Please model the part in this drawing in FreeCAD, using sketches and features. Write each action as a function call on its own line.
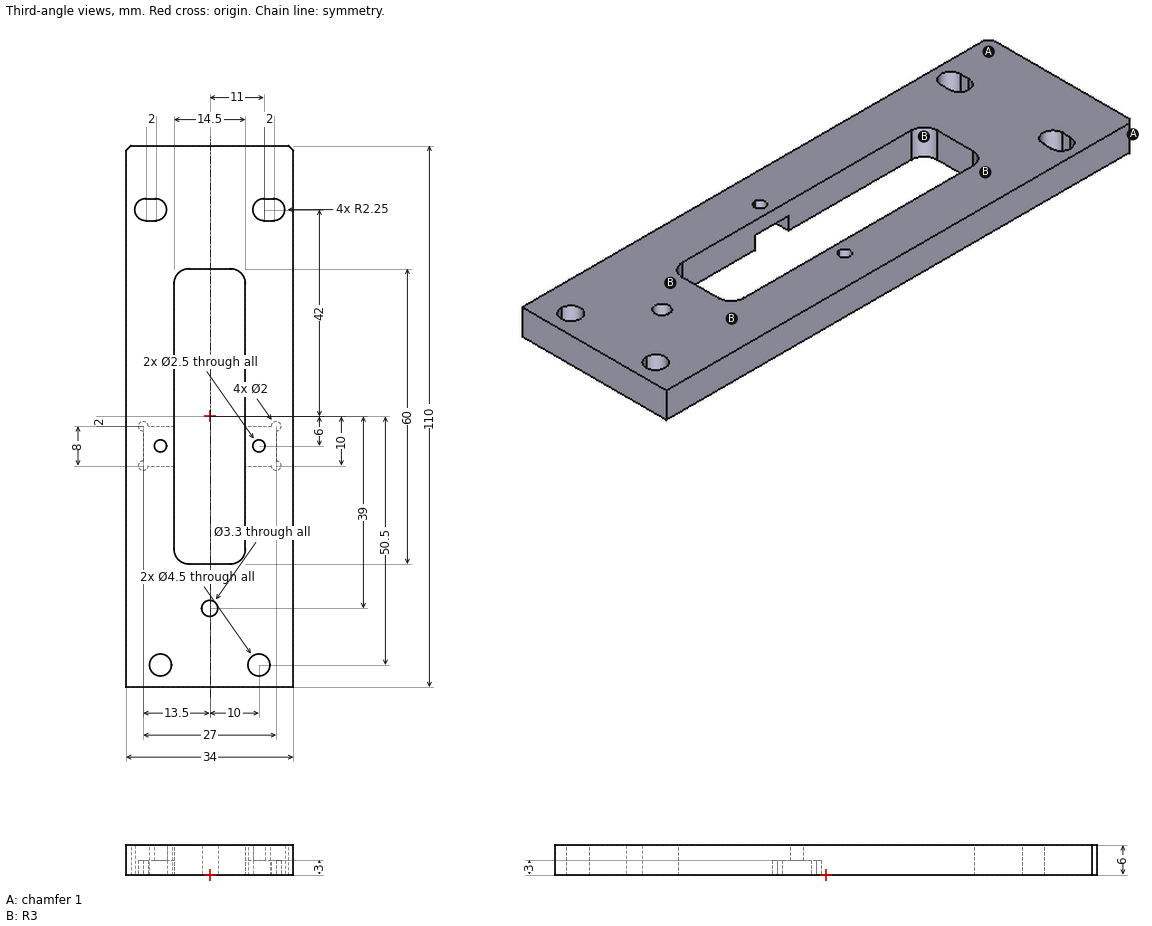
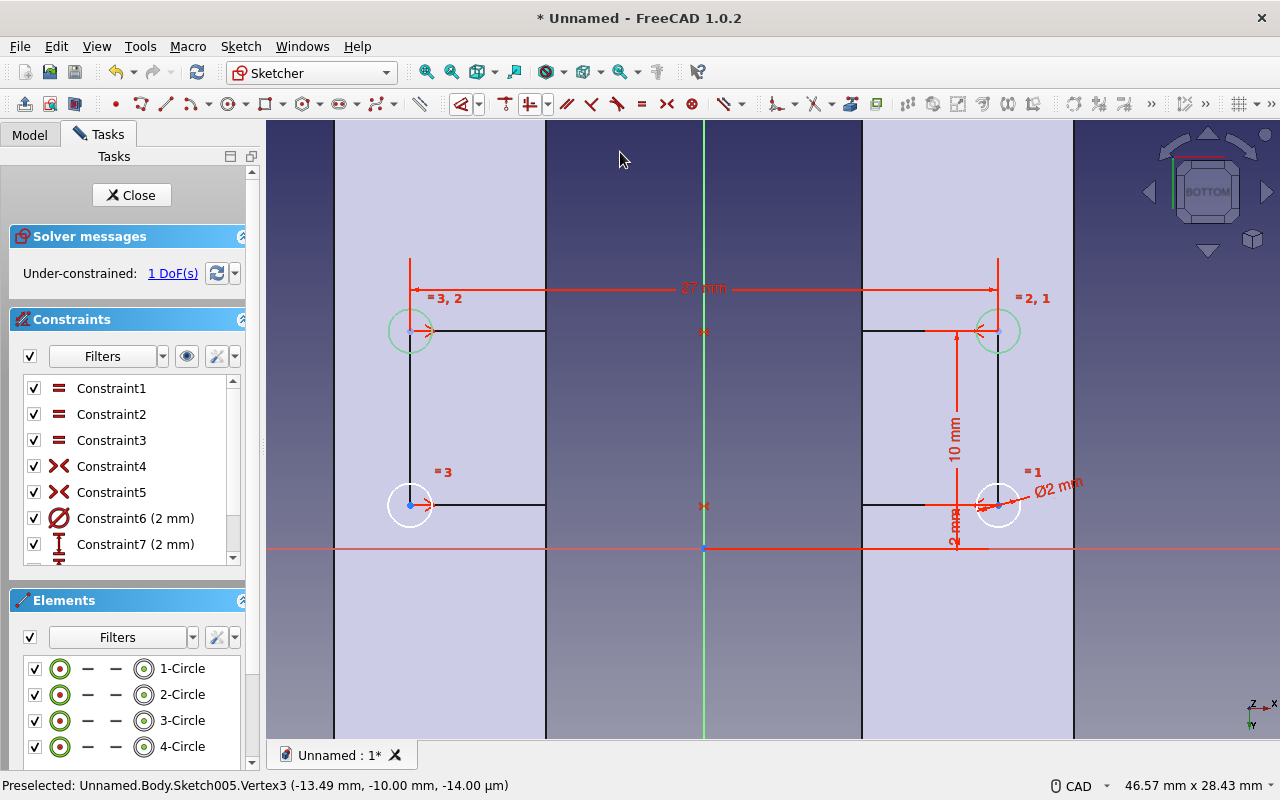
click(998, 505)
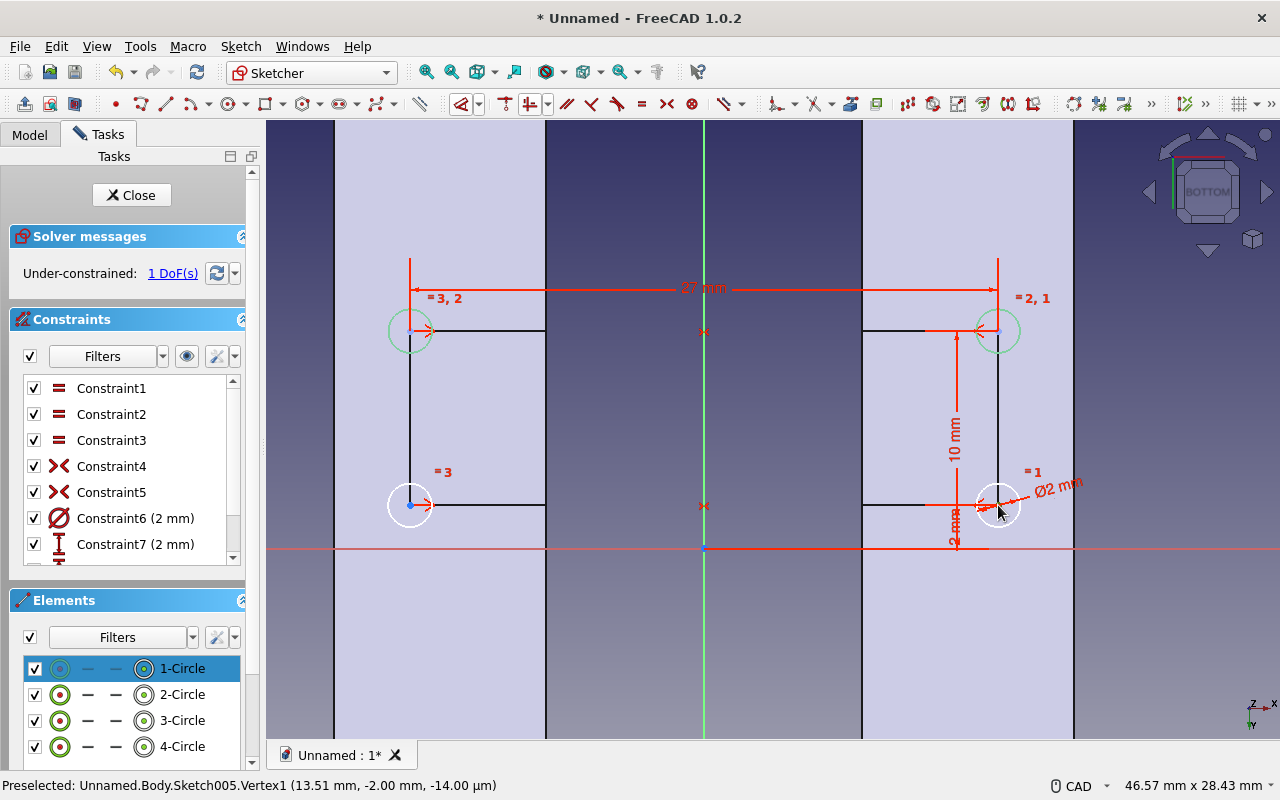
click(410, 331)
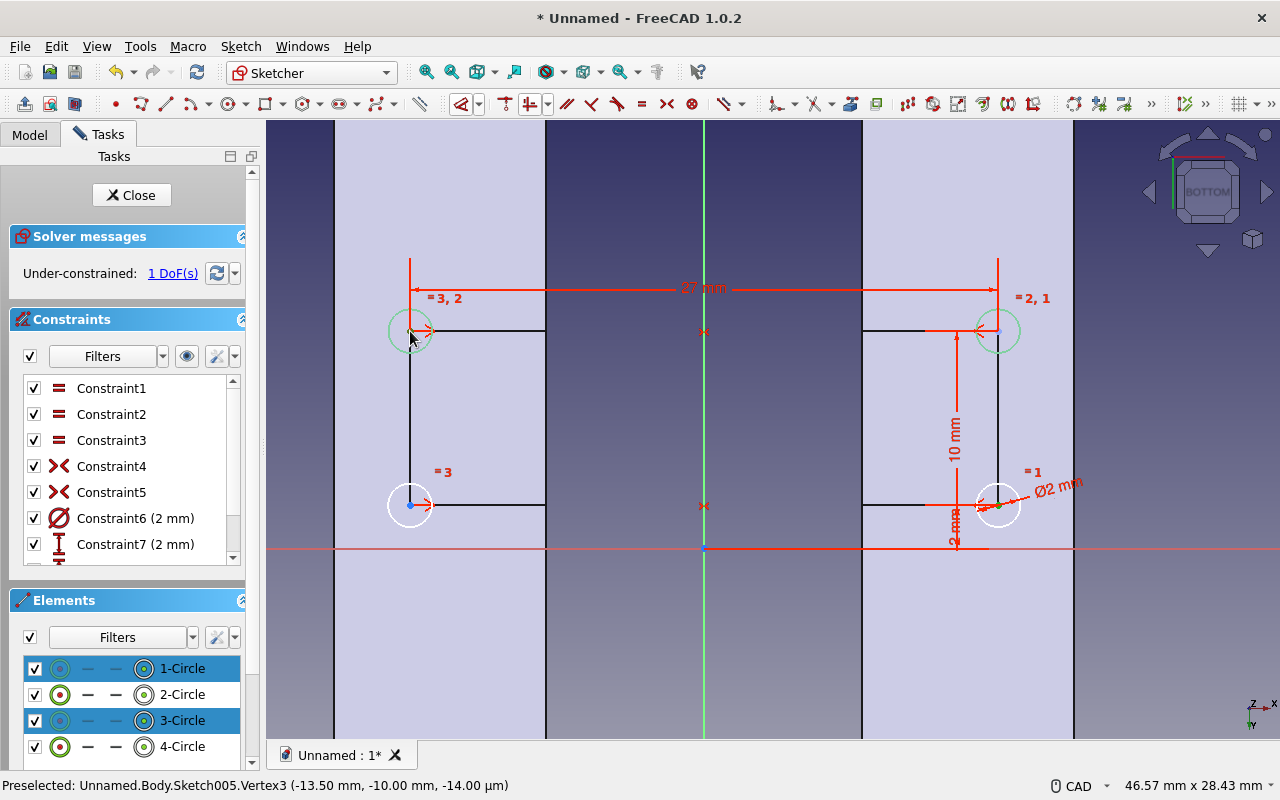
click(478, 104)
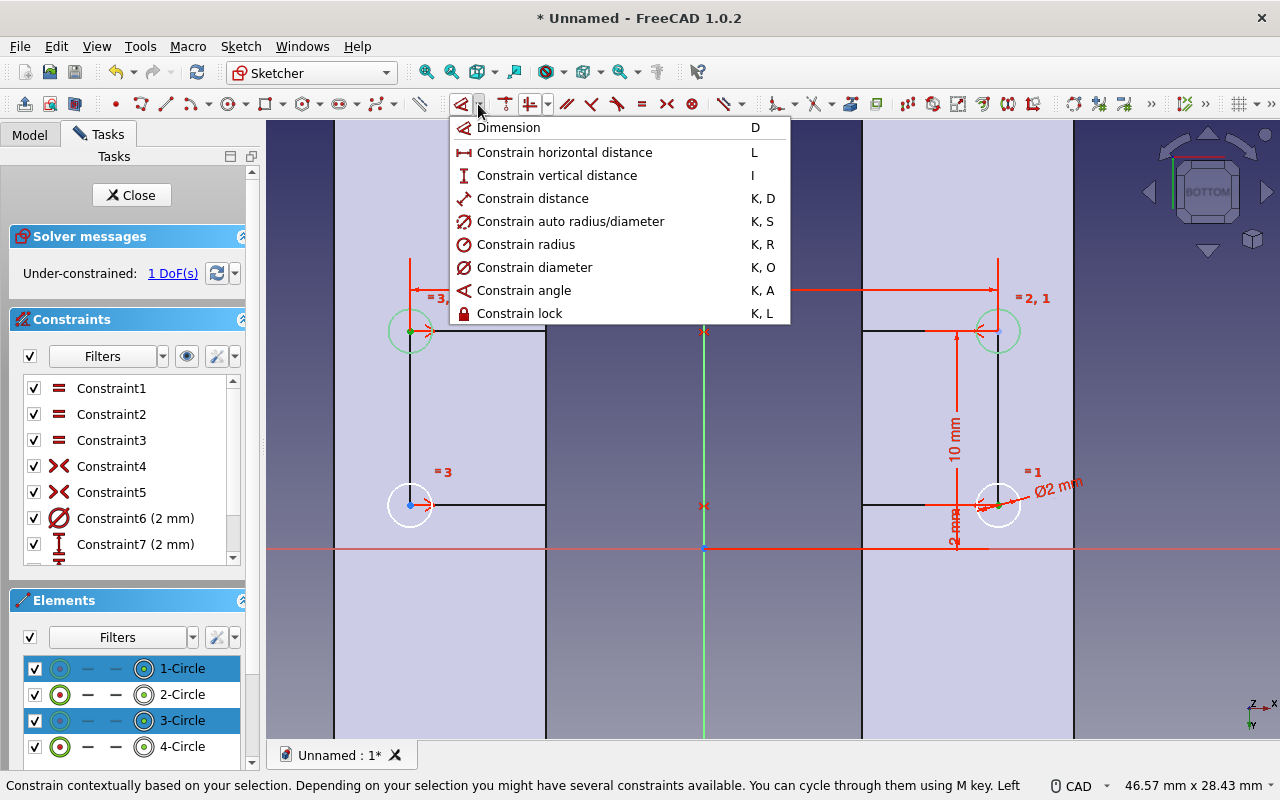
click(620, 152)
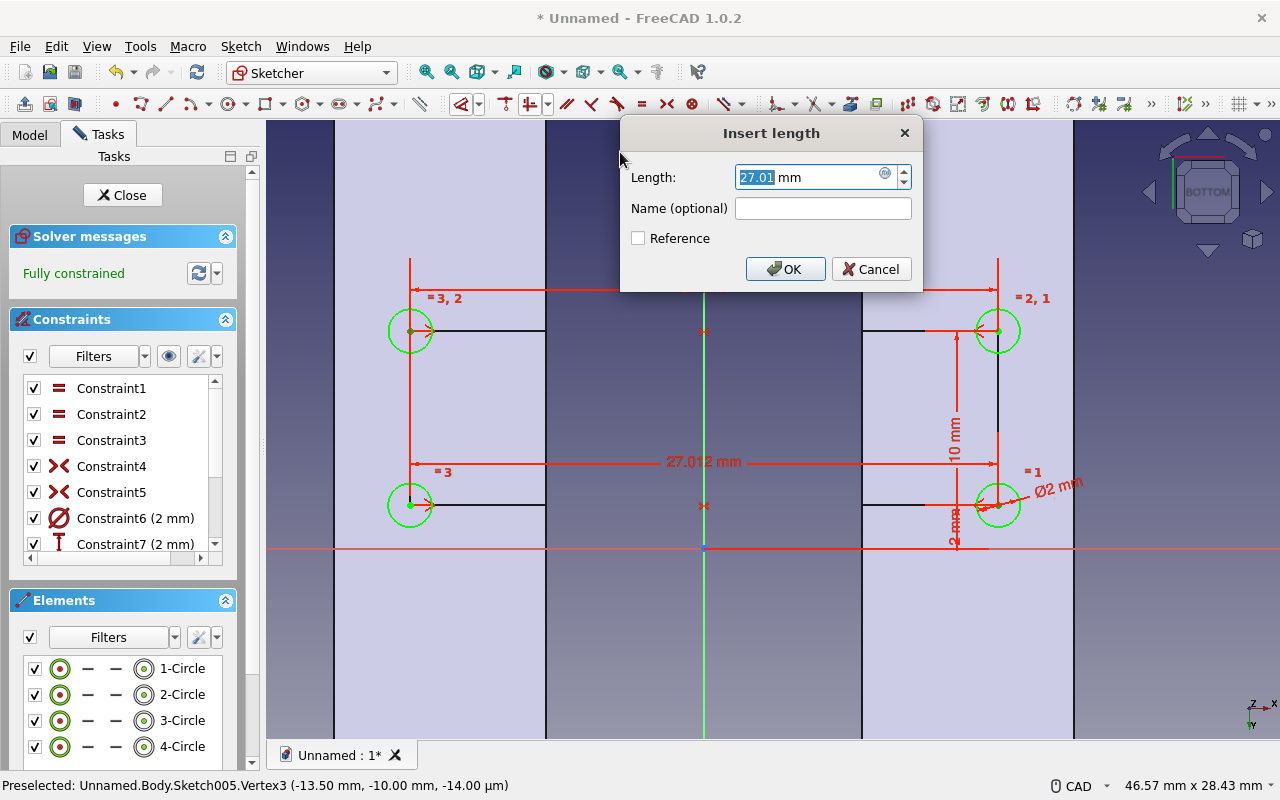
text(27)
key(Return)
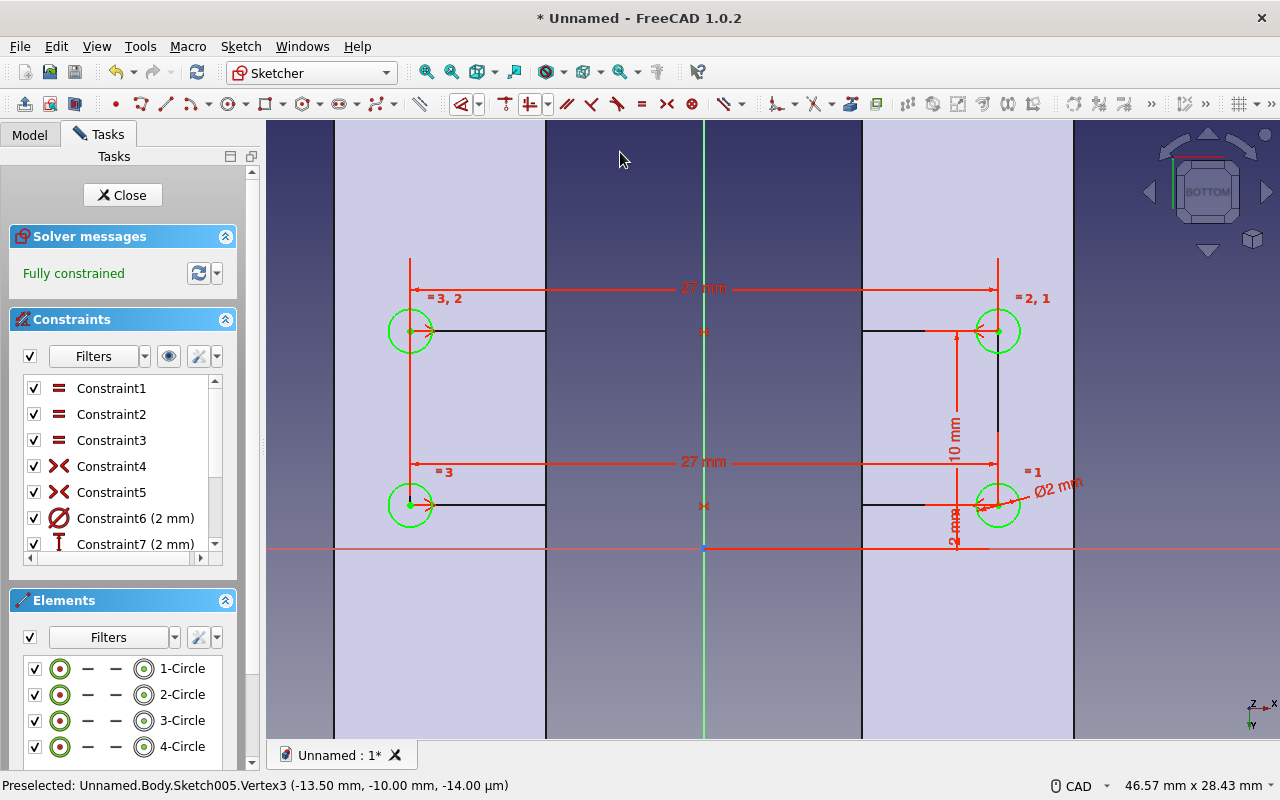
click(123, 195)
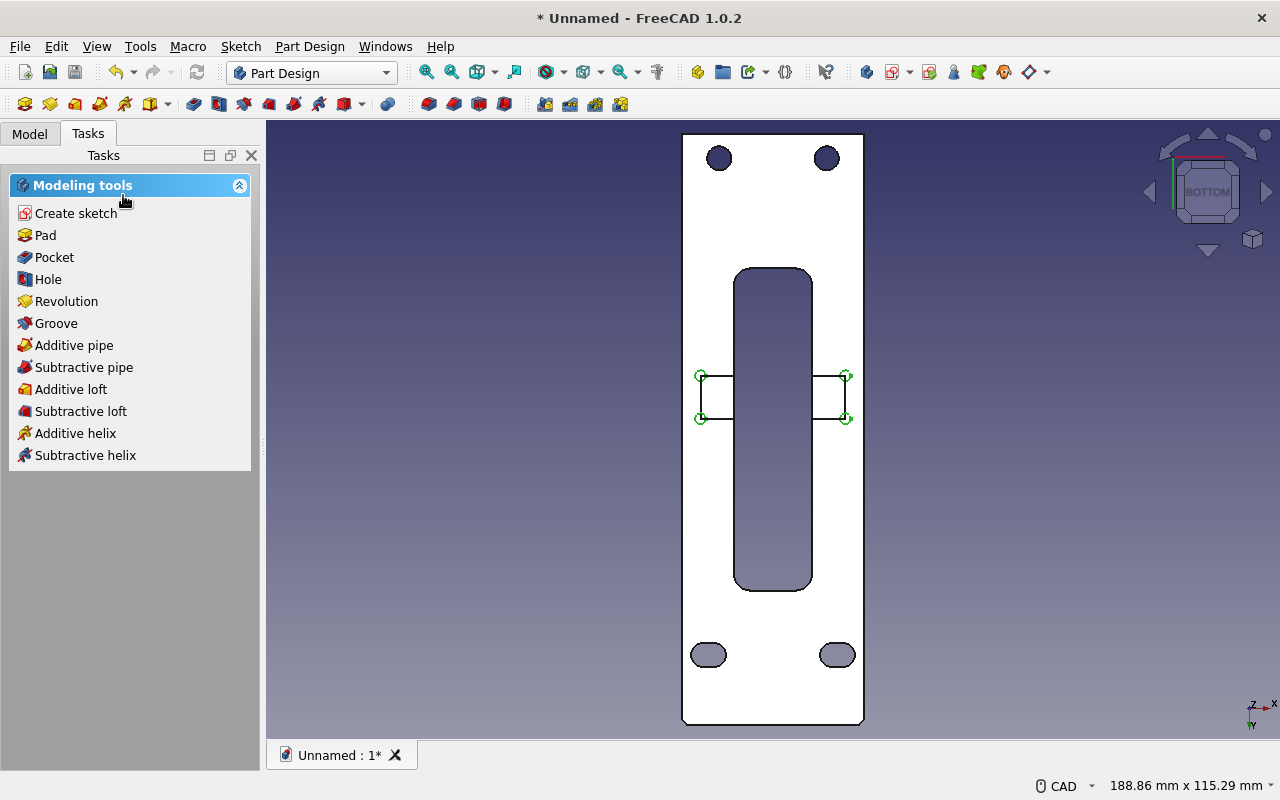
click(194, 104)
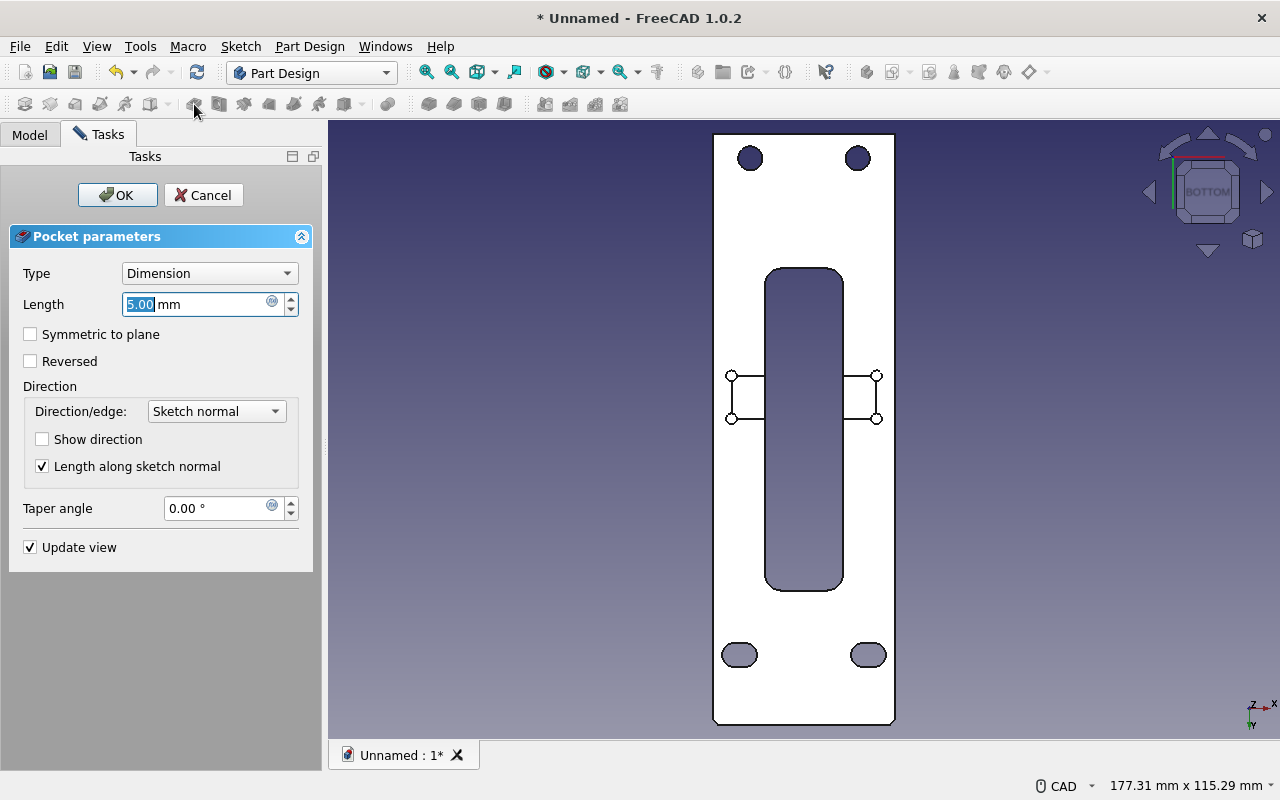
text(3)
key(Tab)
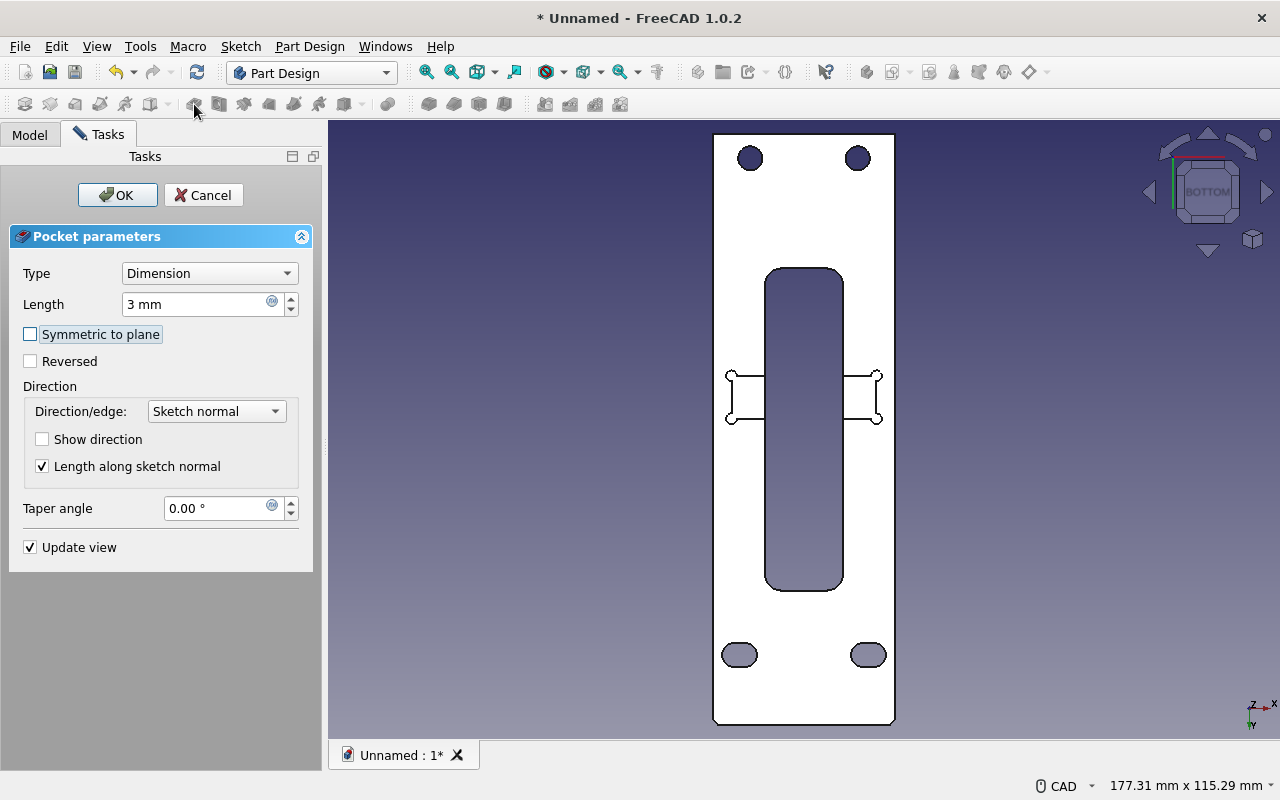
click(118, 195)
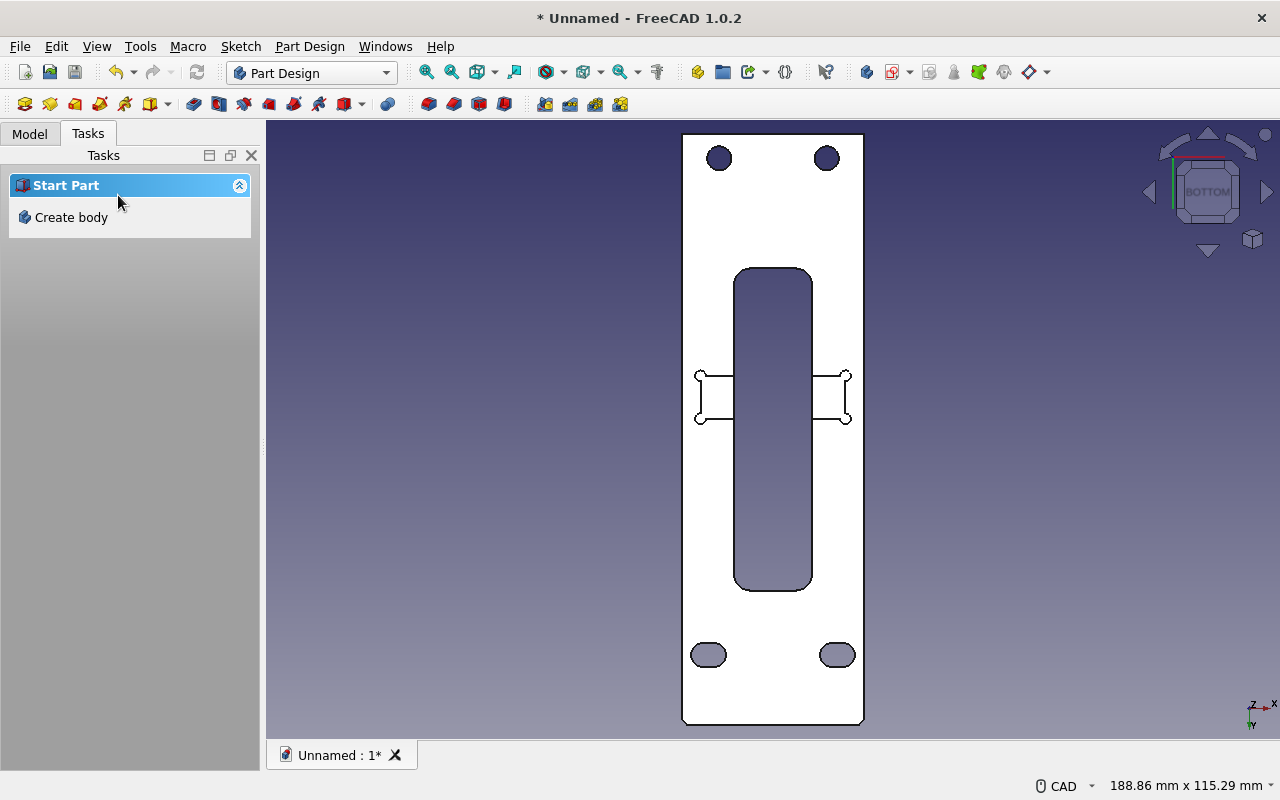
click(773, 682)